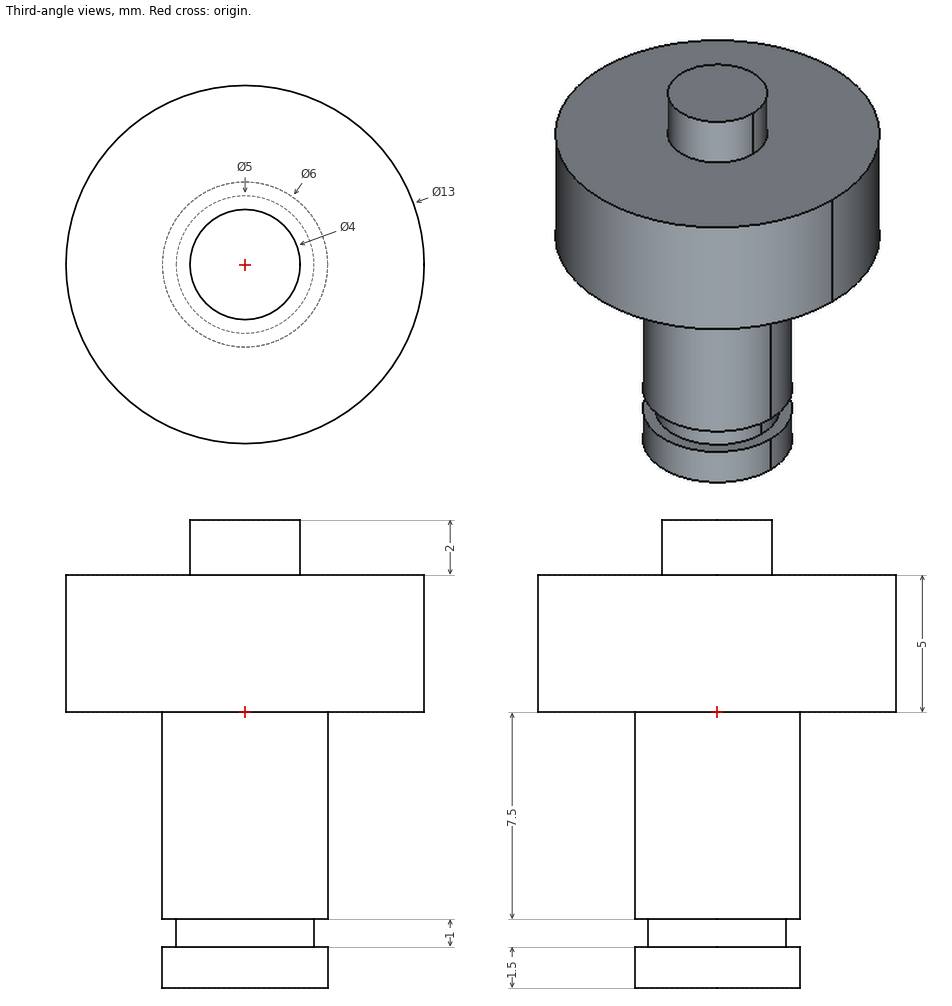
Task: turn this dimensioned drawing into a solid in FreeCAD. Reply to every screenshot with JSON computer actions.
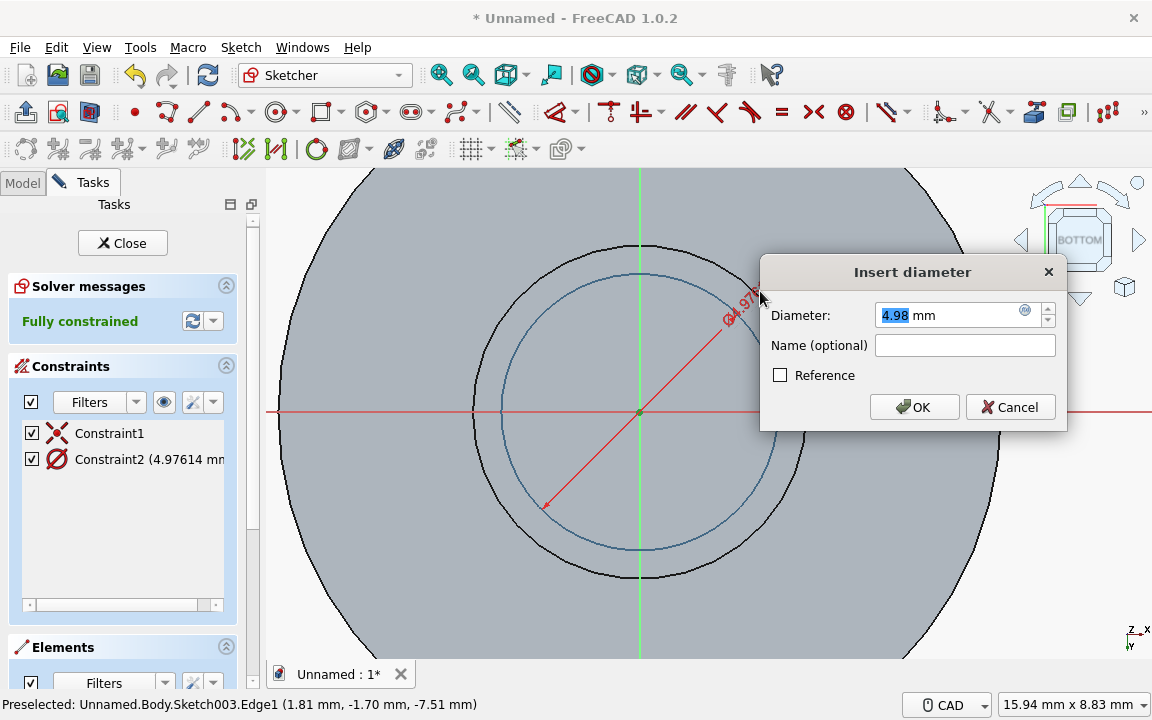
{"action": "type", "text": "5"}
{"action": "key", "text": "Return"}
{"action": "key", "text": "Escape"}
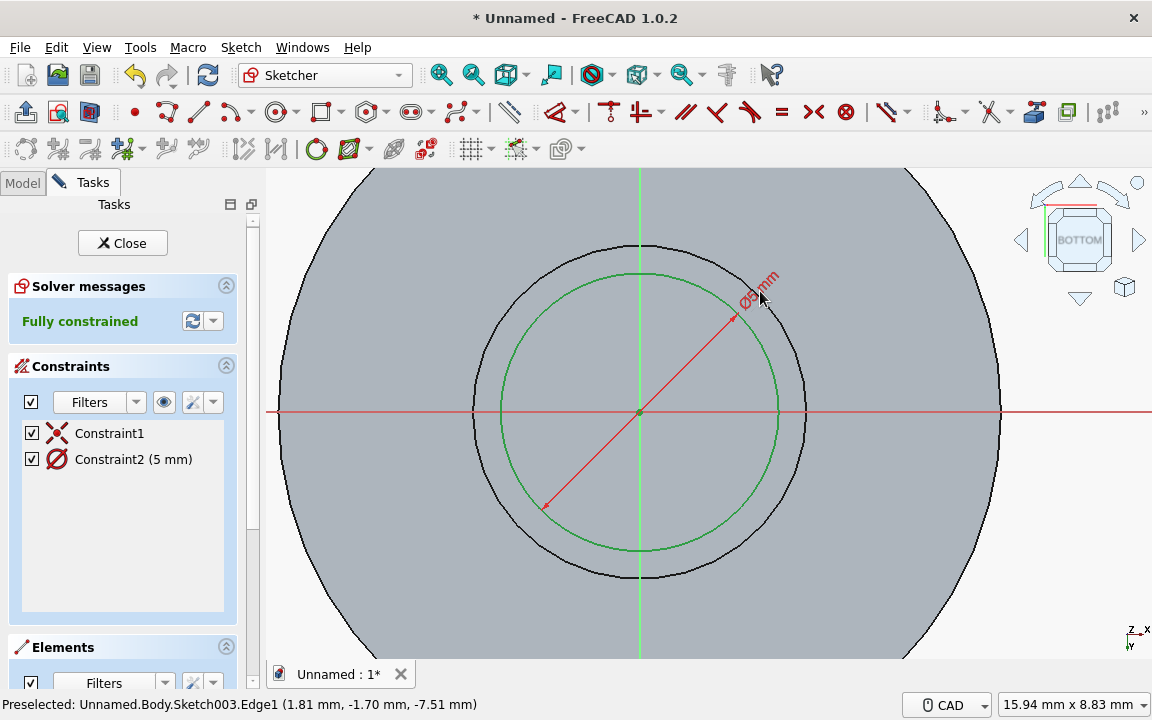
{"action": "left_click", "coordinate": [123, 243]}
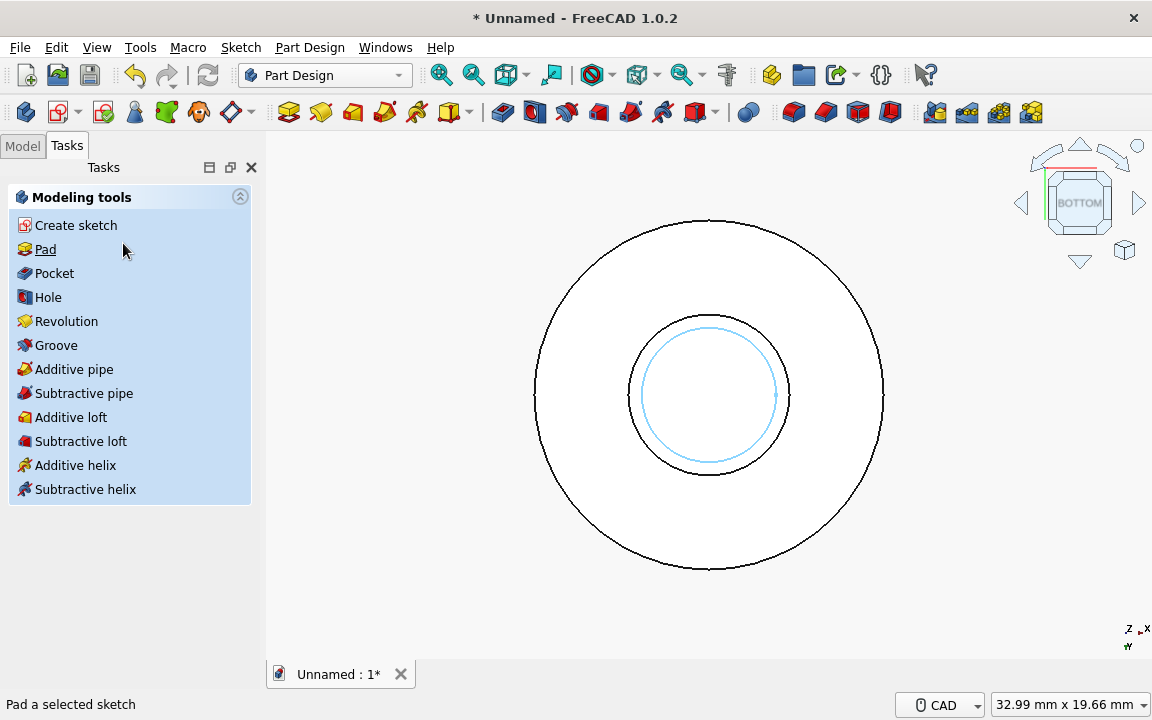
{"action": "left_click", "coordinate": [290, 112]}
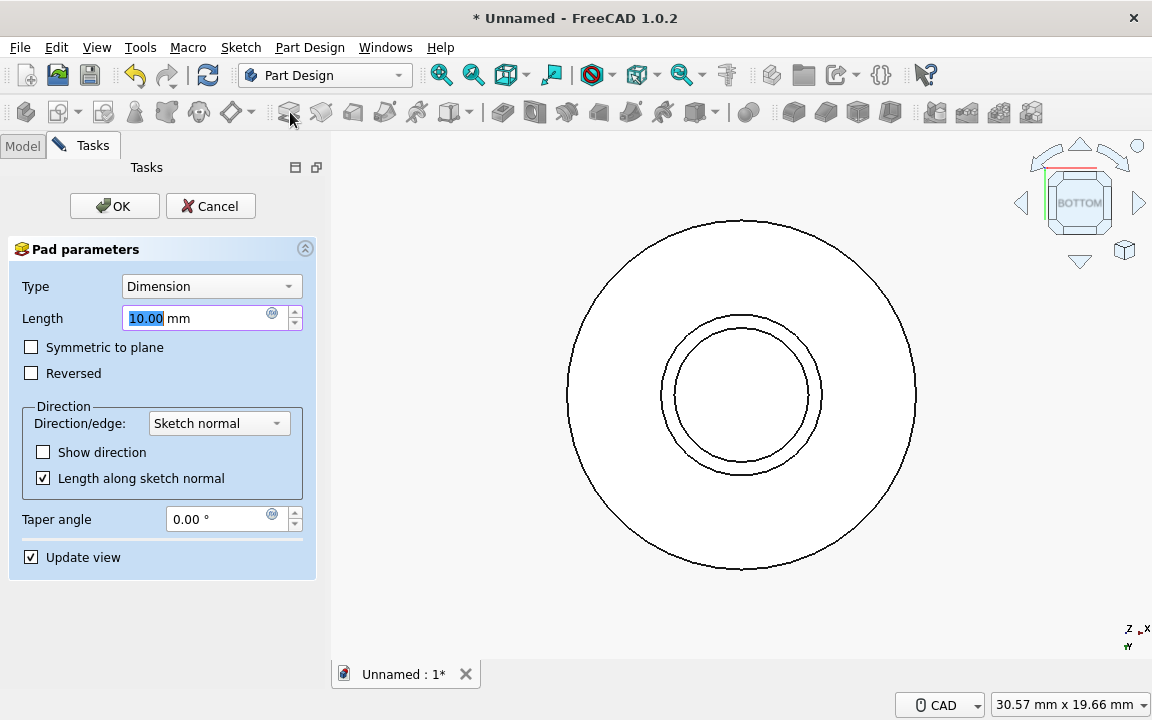
{"action": "type", "text": "1"}
{"action": "key", "text": "Tab"}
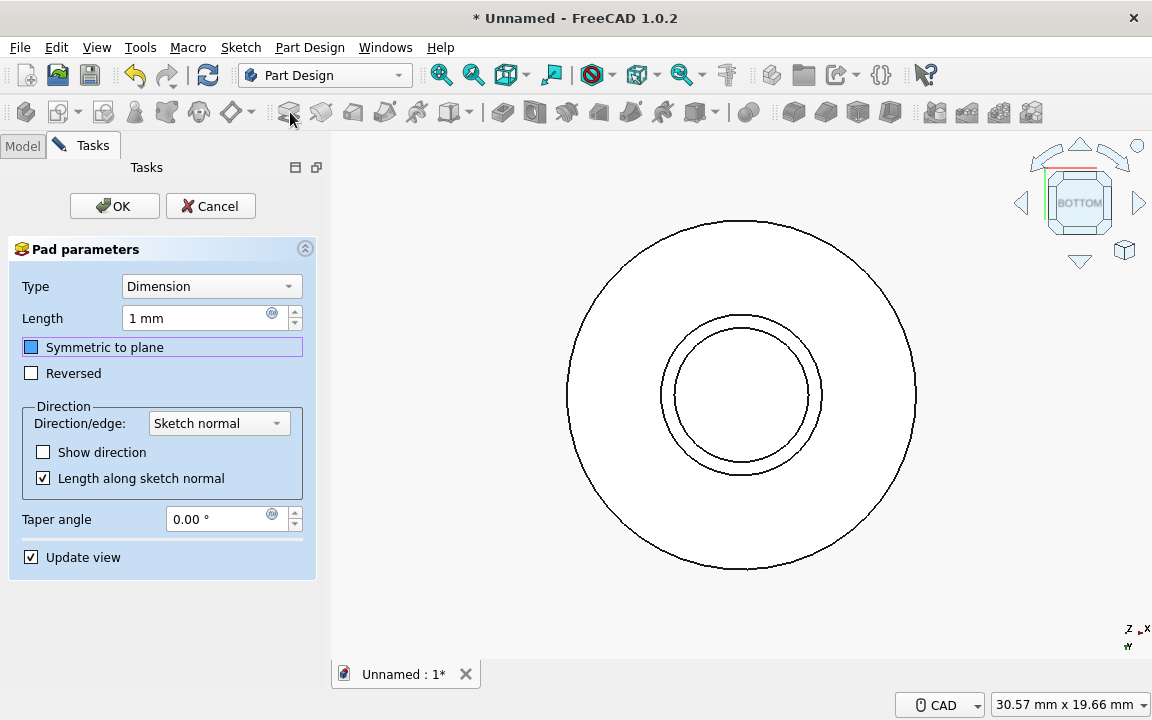
{"action": "left_click", "coordinate": [115, 206]}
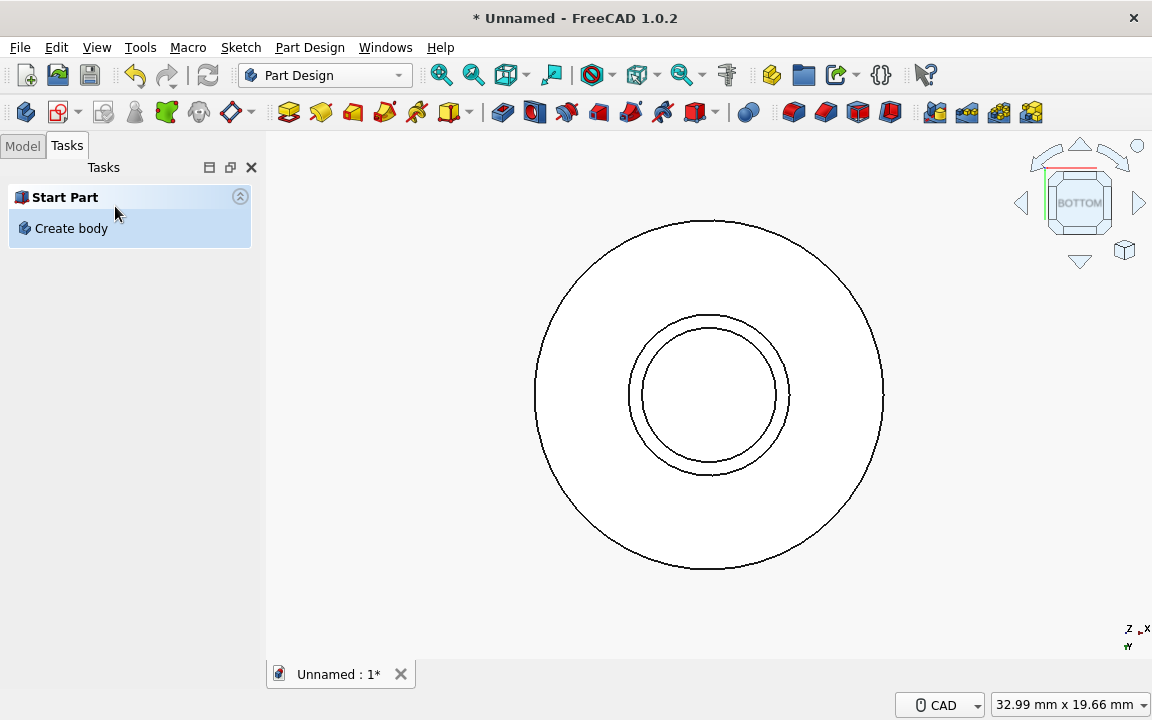
{"action": "left_click", "coordinate": [709, 394]}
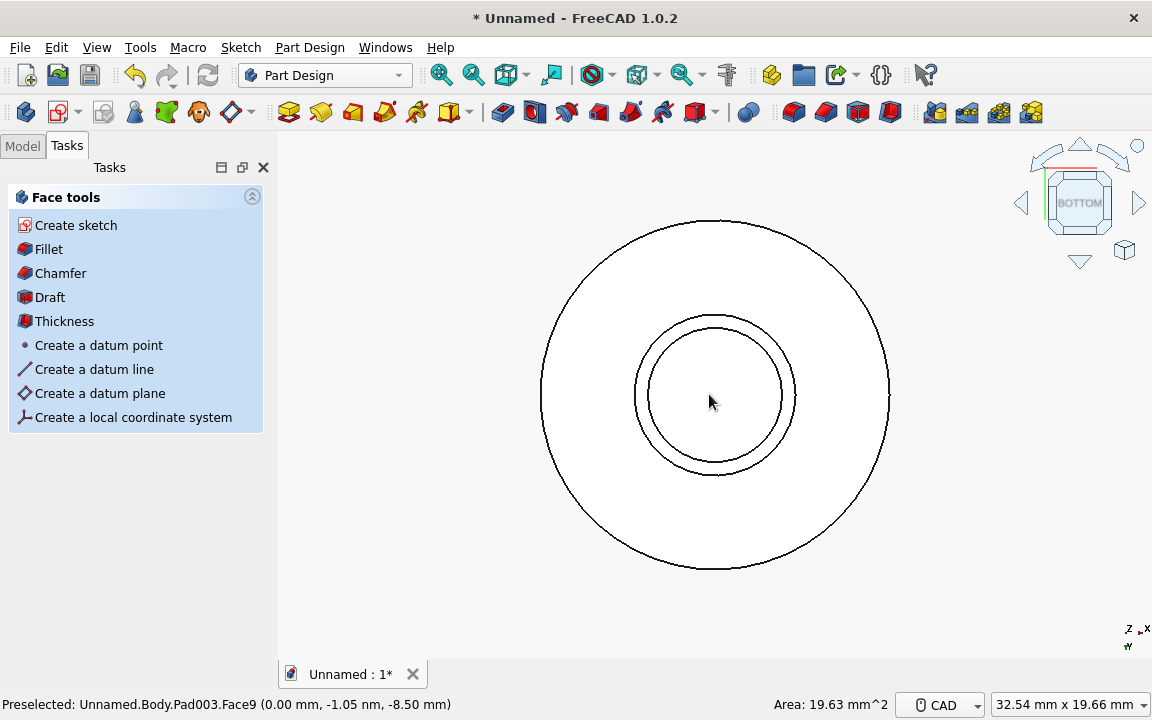
{"action": "left_click", "coordinate": [58, 112]}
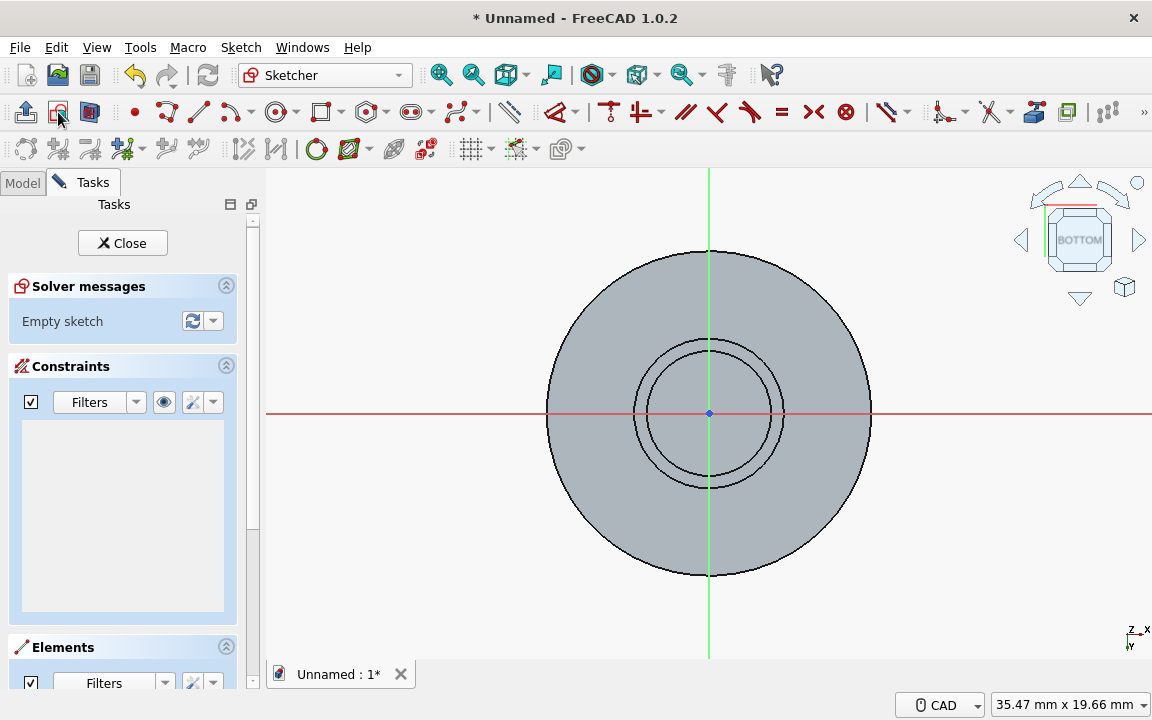
{"action": "scroll", "coordinate": [765, 414], "scroll_direction": "up", "scroll_amount": 4}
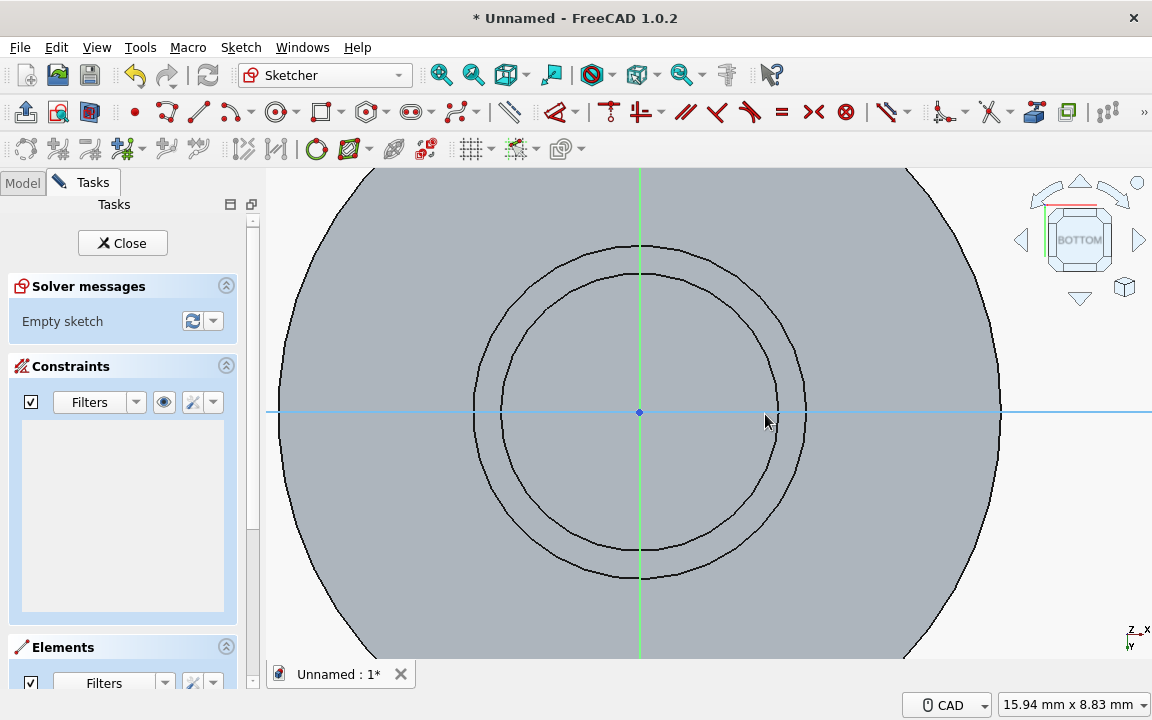
{"action": "left_click", "coordinate": [276, 112]}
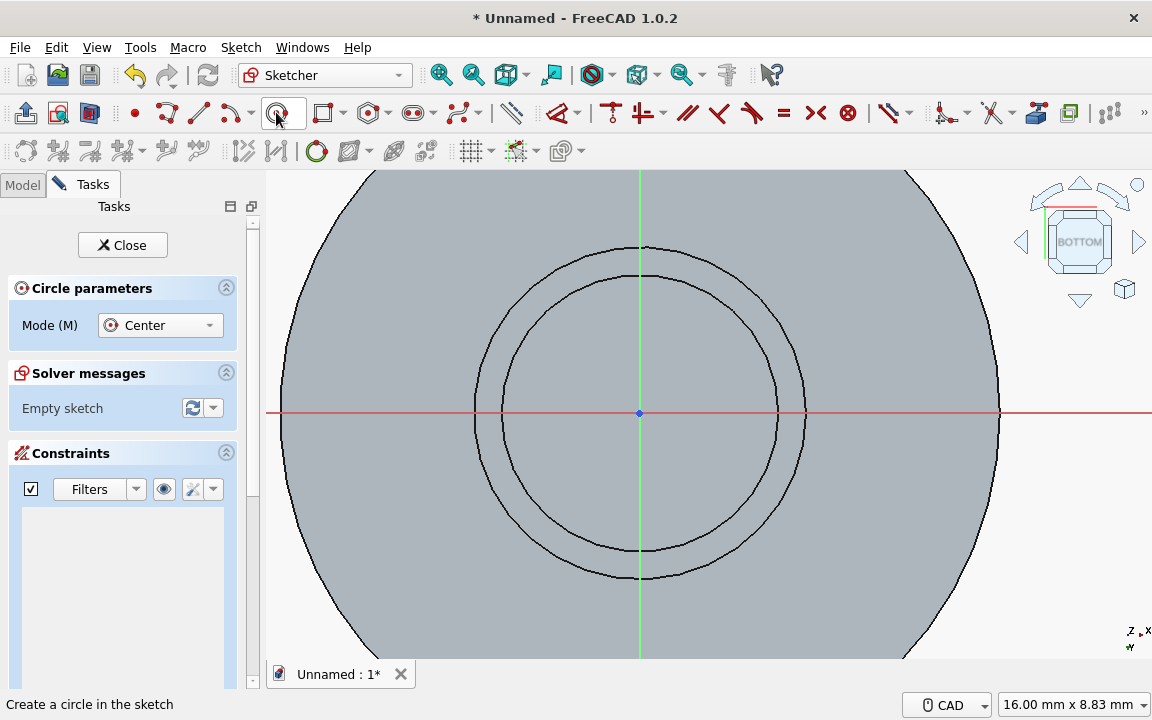
{"action": "left_click", "coordinate": [640, 413]}
{"action": "left_click", "coordinate": [757, 296]}
{"action": "key", "text": "Escape"}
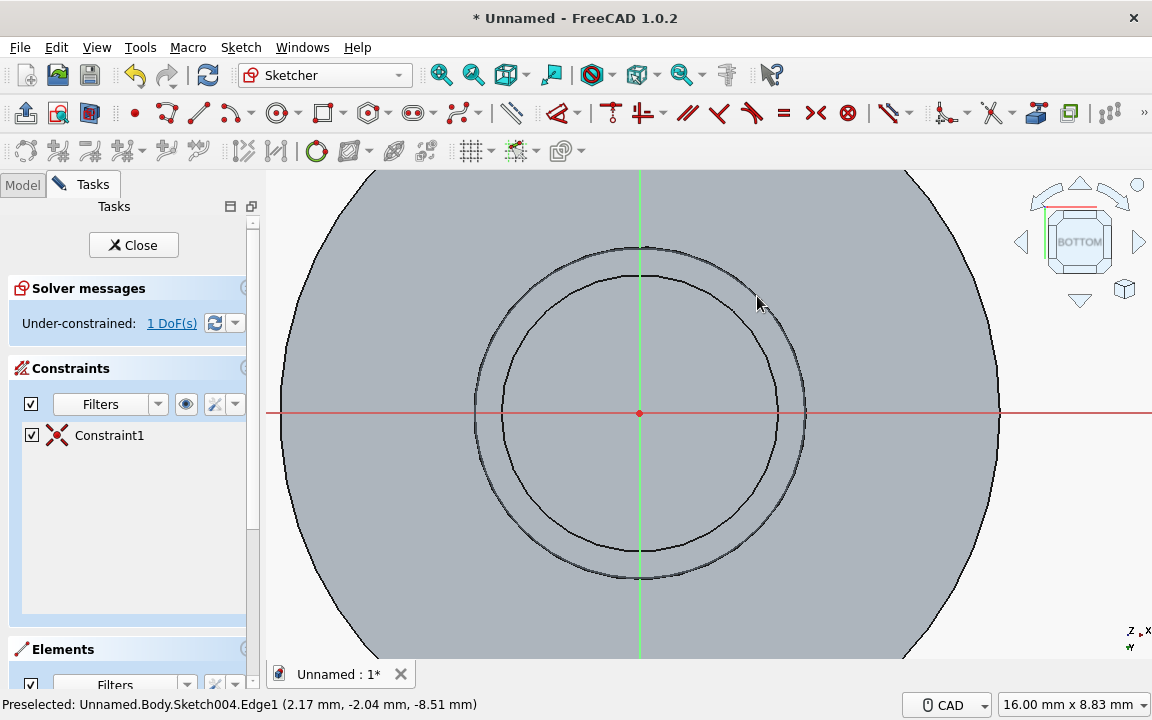
{"action": "key", "text": "d"}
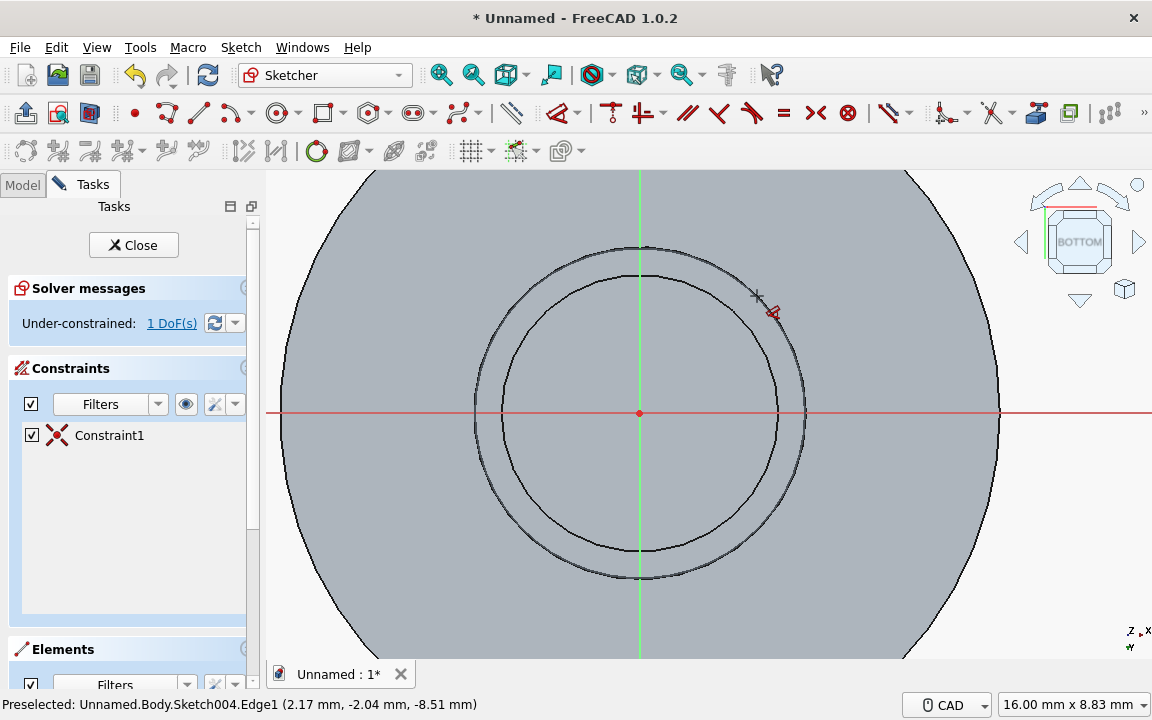
{"action": "left_click", "coordinate": [756, 296]}
{"action": "left_click", "coordinate": [779, 273]}